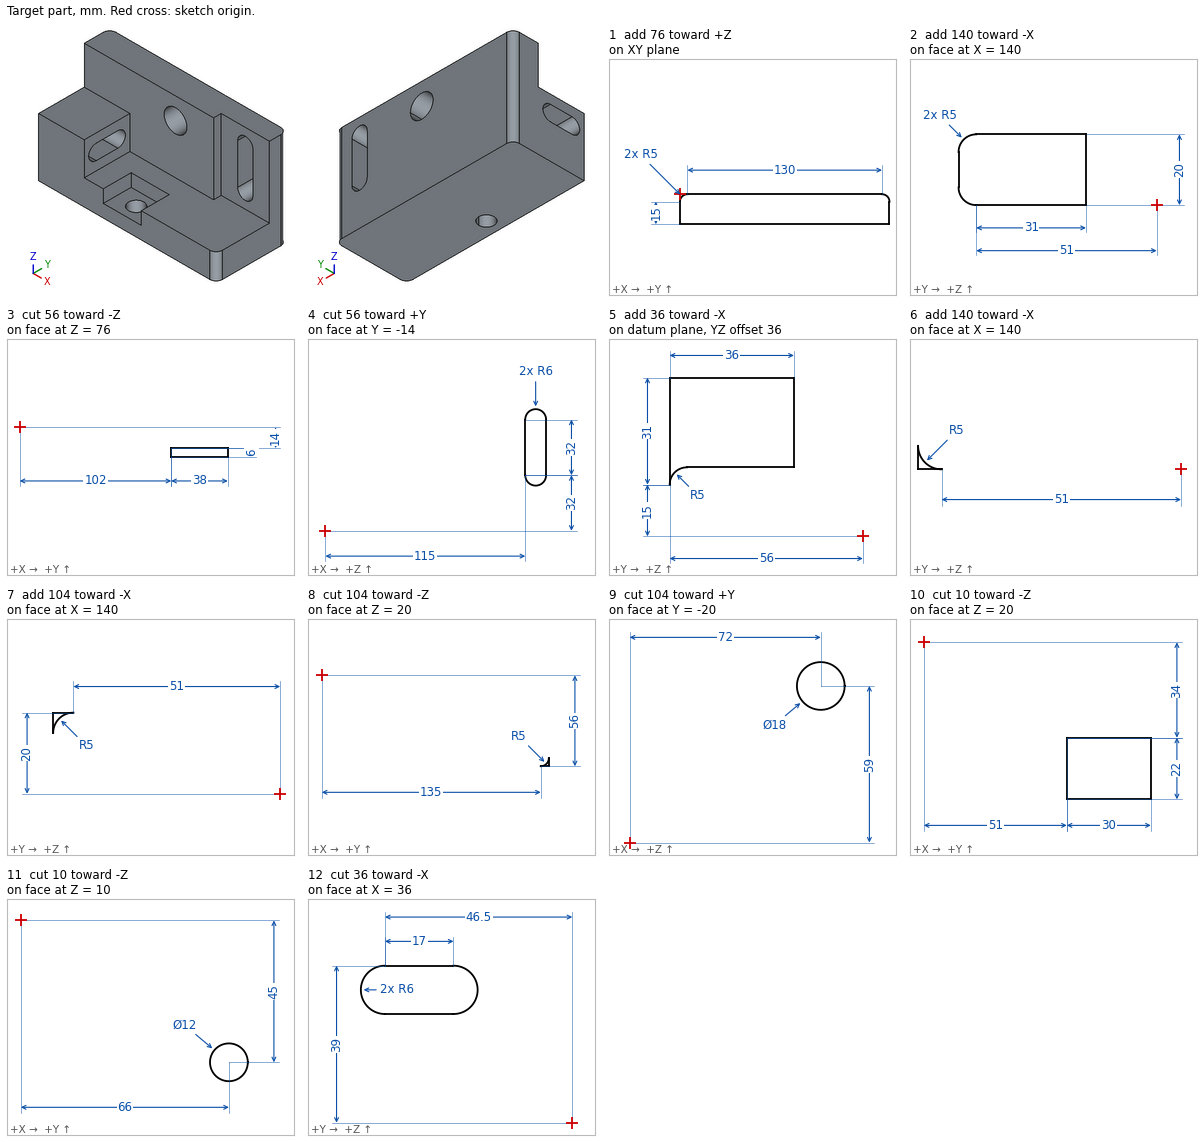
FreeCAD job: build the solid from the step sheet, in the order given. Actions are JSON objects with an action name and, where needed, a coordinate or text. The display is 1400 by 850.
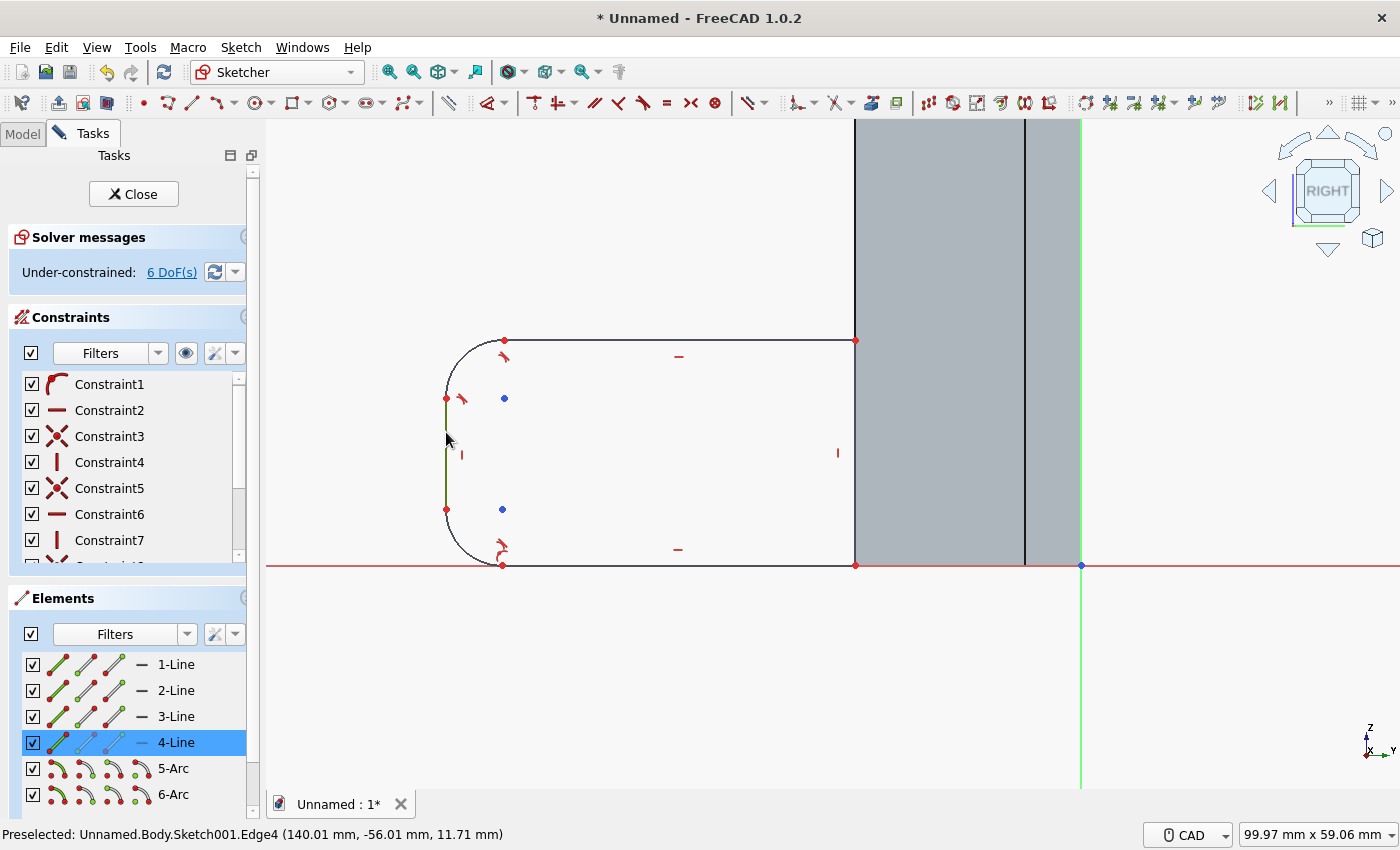
{"action": "left_click", "coordinate": [452, 535]}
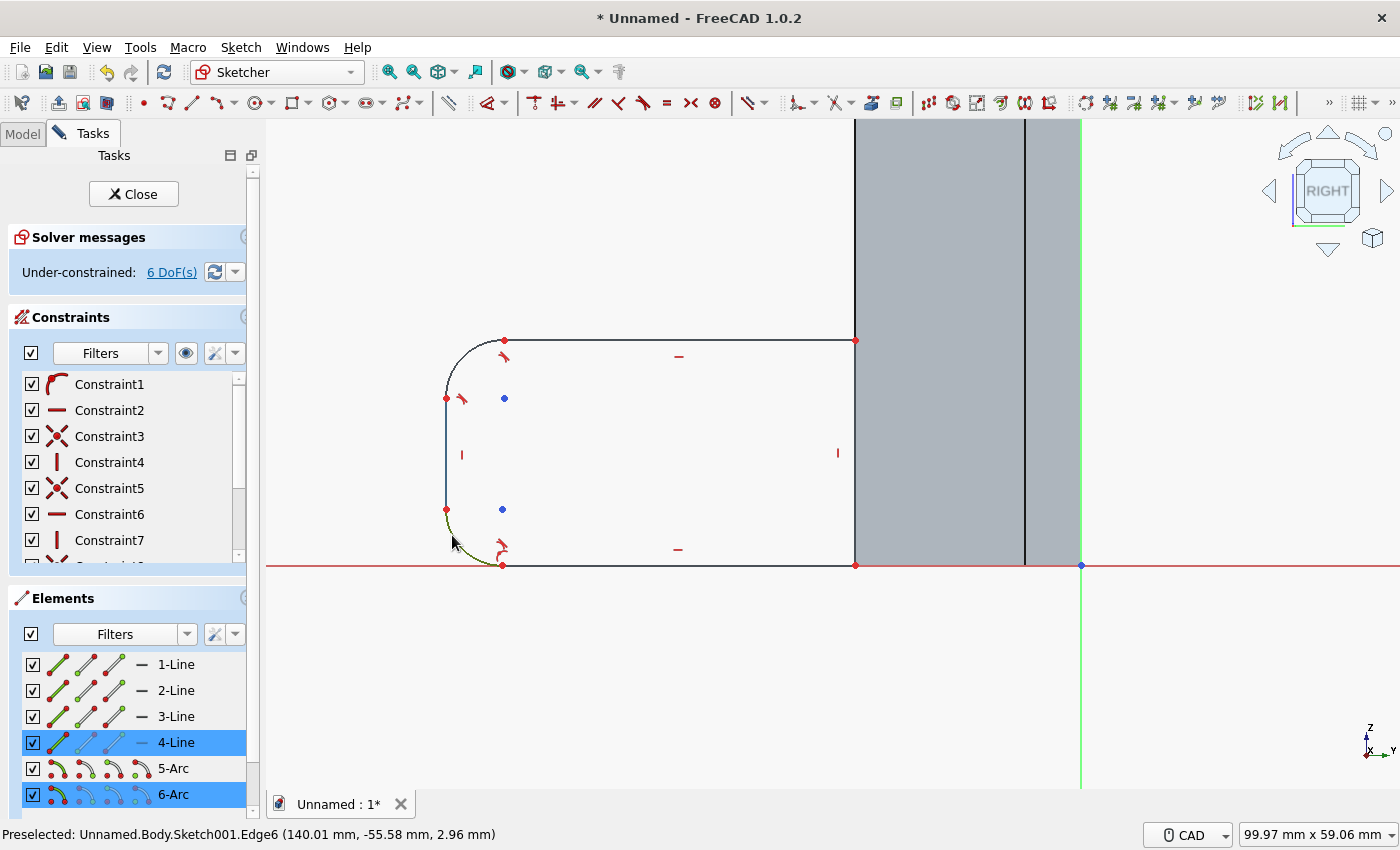
{"action": "left_click", "coordinate": [644, 104]}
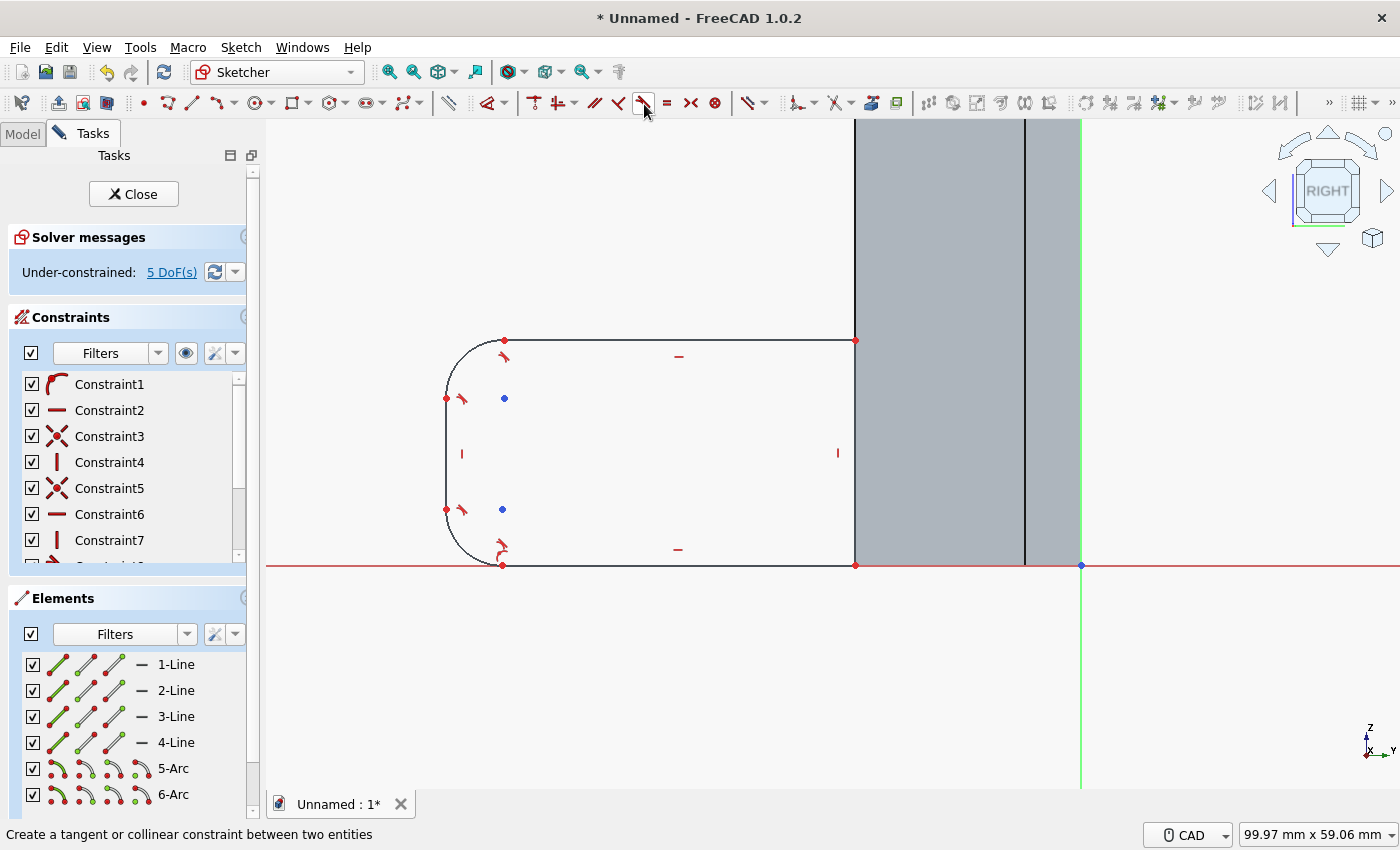
{"action": "left_click", "coordinate": [478, 346]}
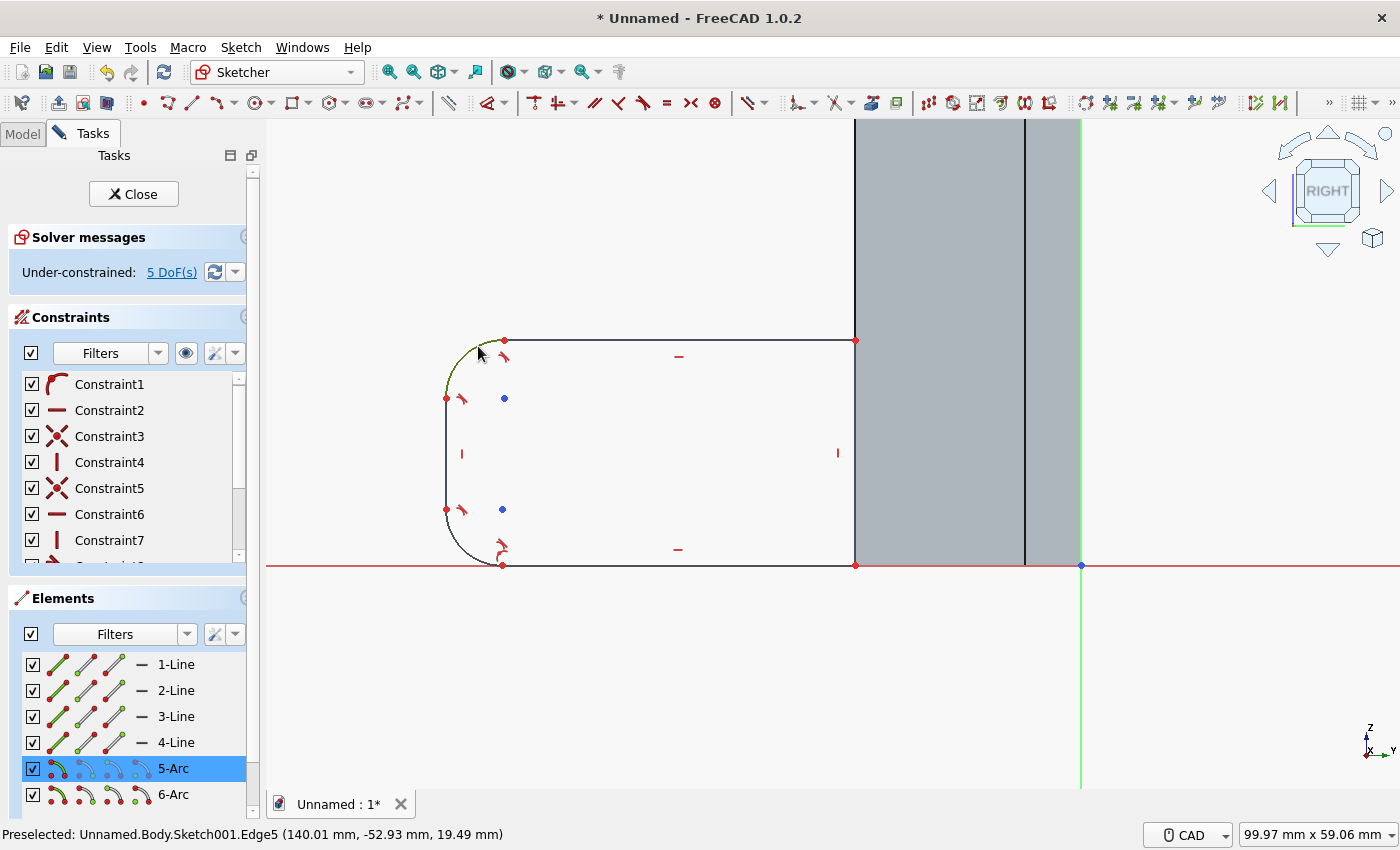
{"action": "left_click", "coordinate": [452, 535]}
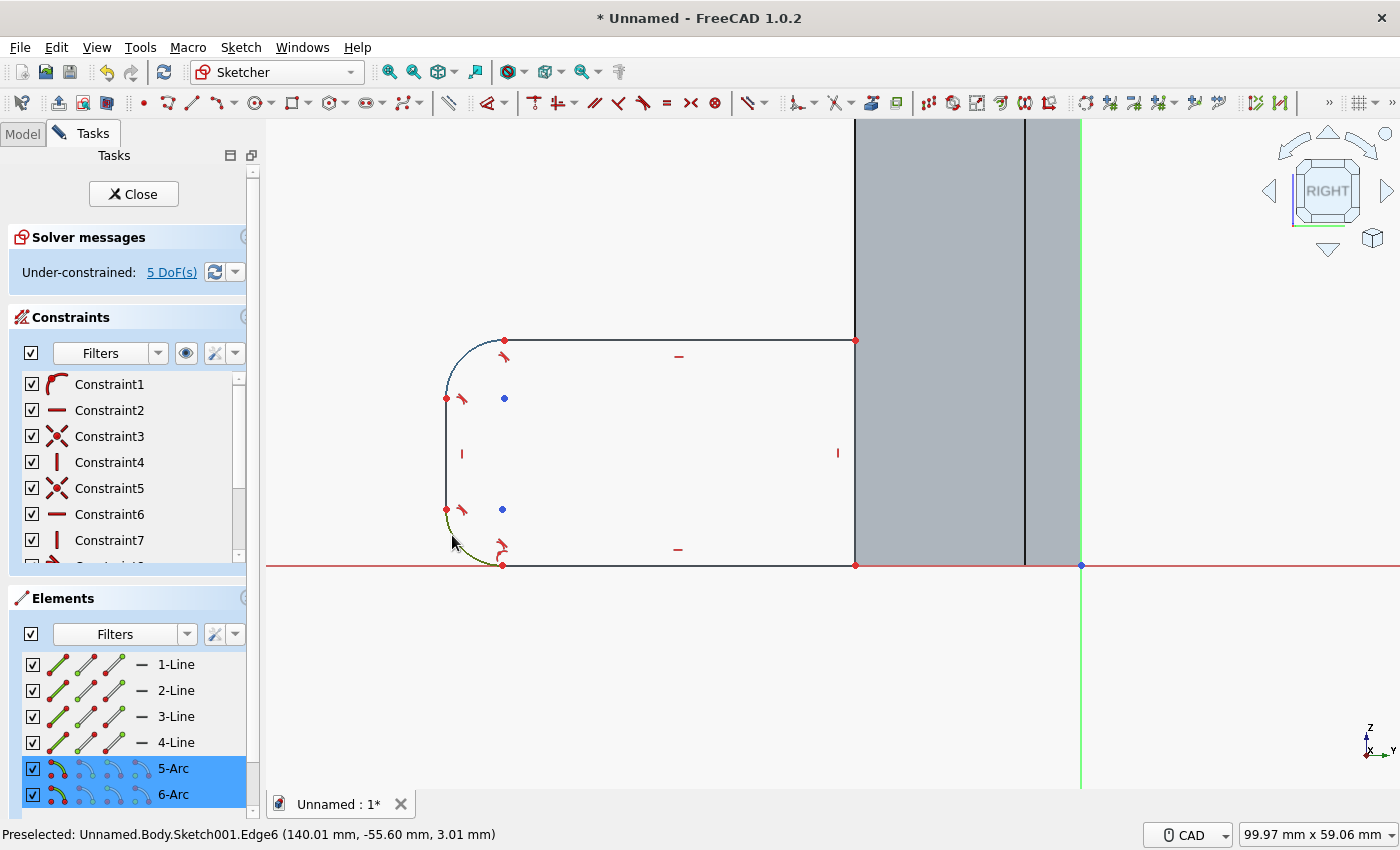
{"action": "left_click", "coordinate": [668, 104]}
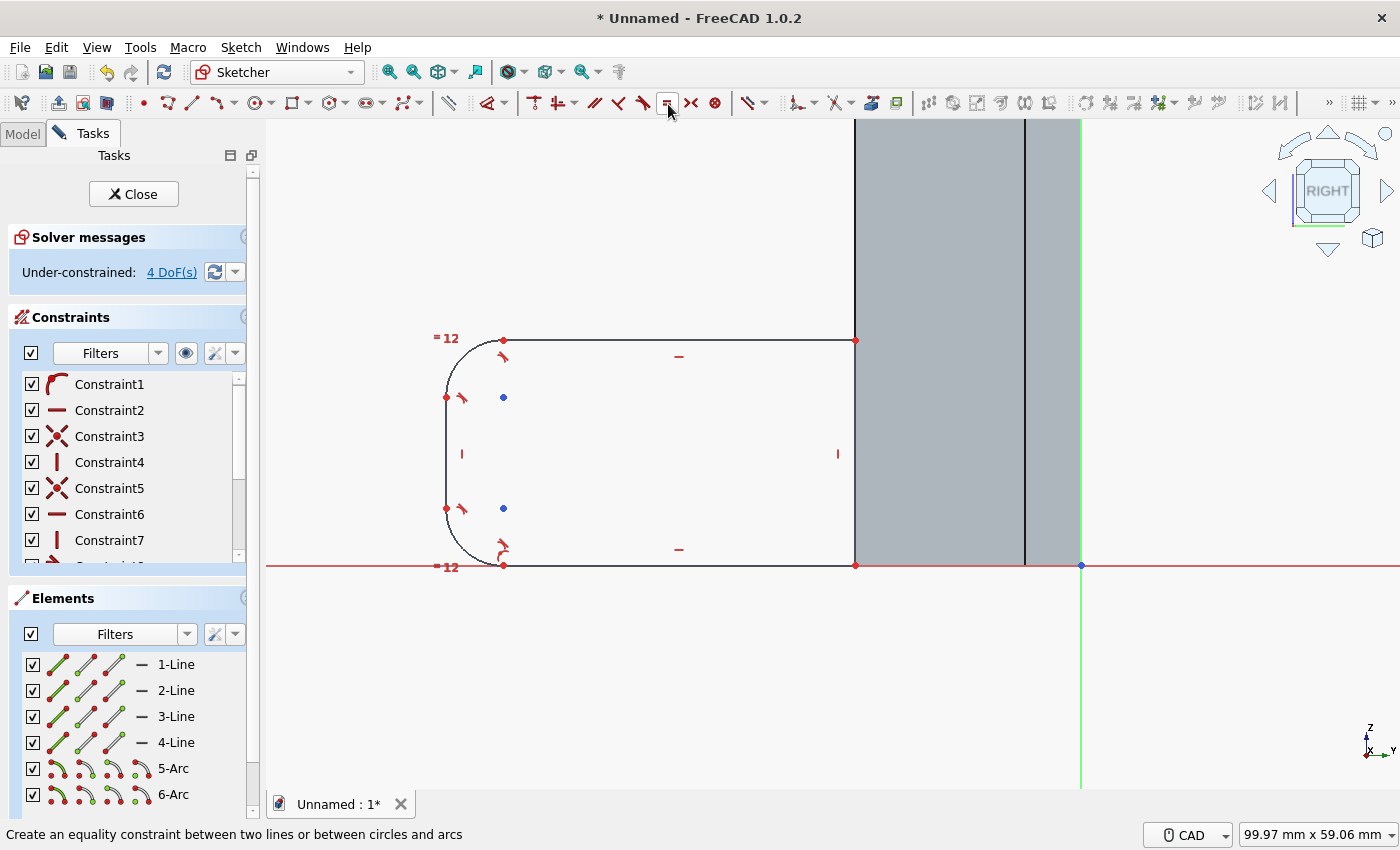
{"action": "key", "text": "d"}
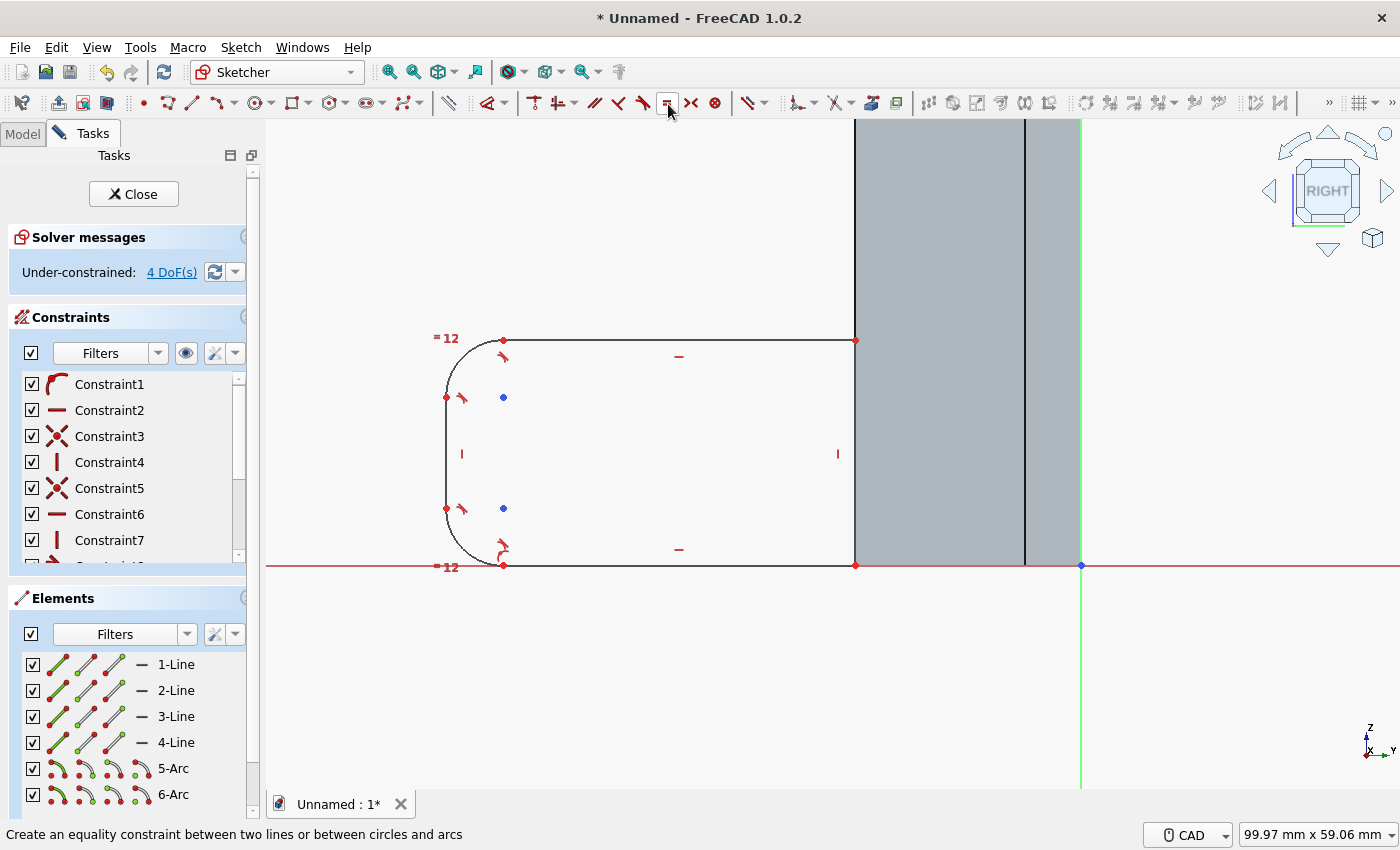
{"action": "left_click", "coordinate": [478, 346]}
{"action": "left_click", "coordinate": [464, 317]}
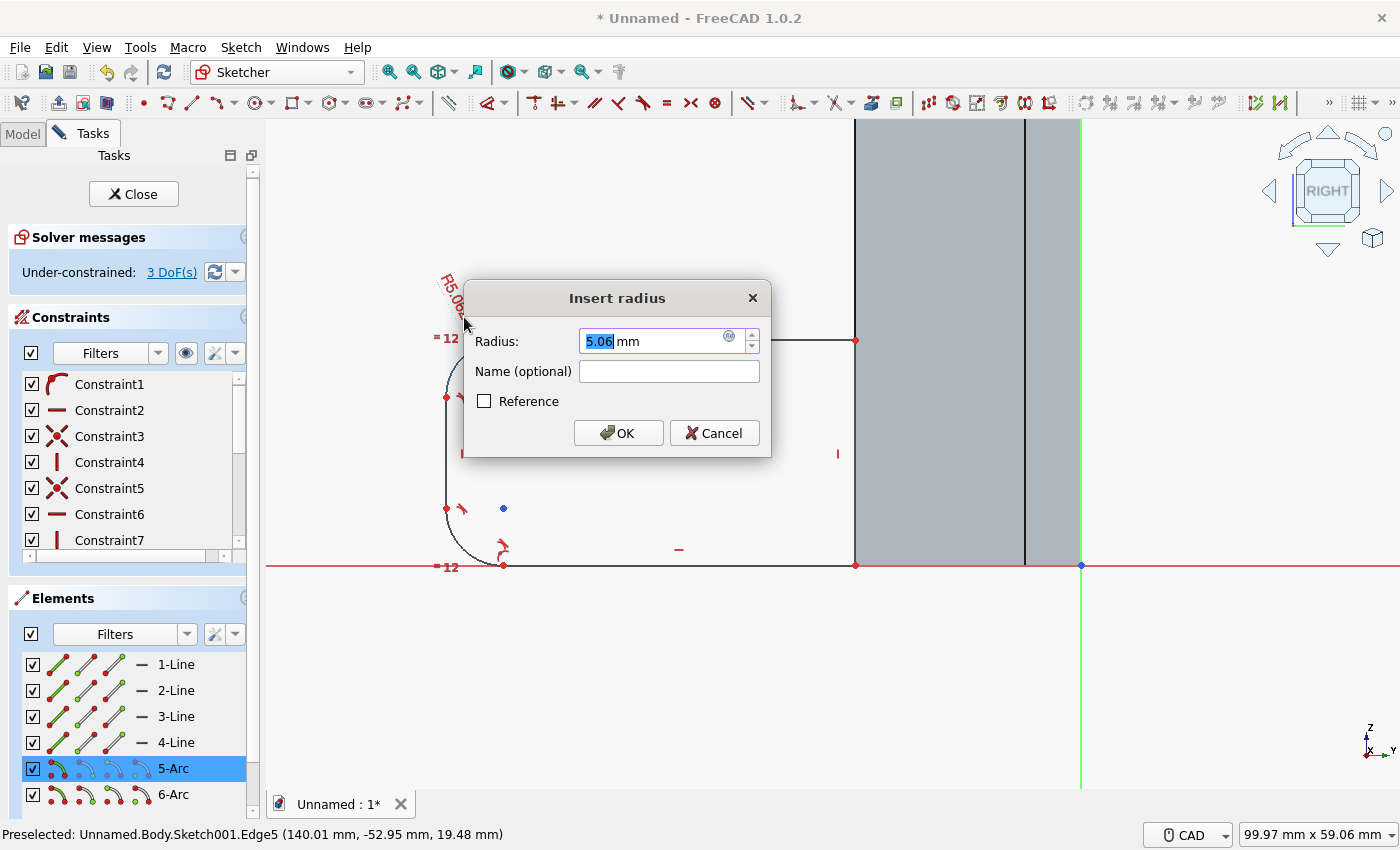
{"action": "type", "text": "5"}
{"action": "key", "text": "Return"}